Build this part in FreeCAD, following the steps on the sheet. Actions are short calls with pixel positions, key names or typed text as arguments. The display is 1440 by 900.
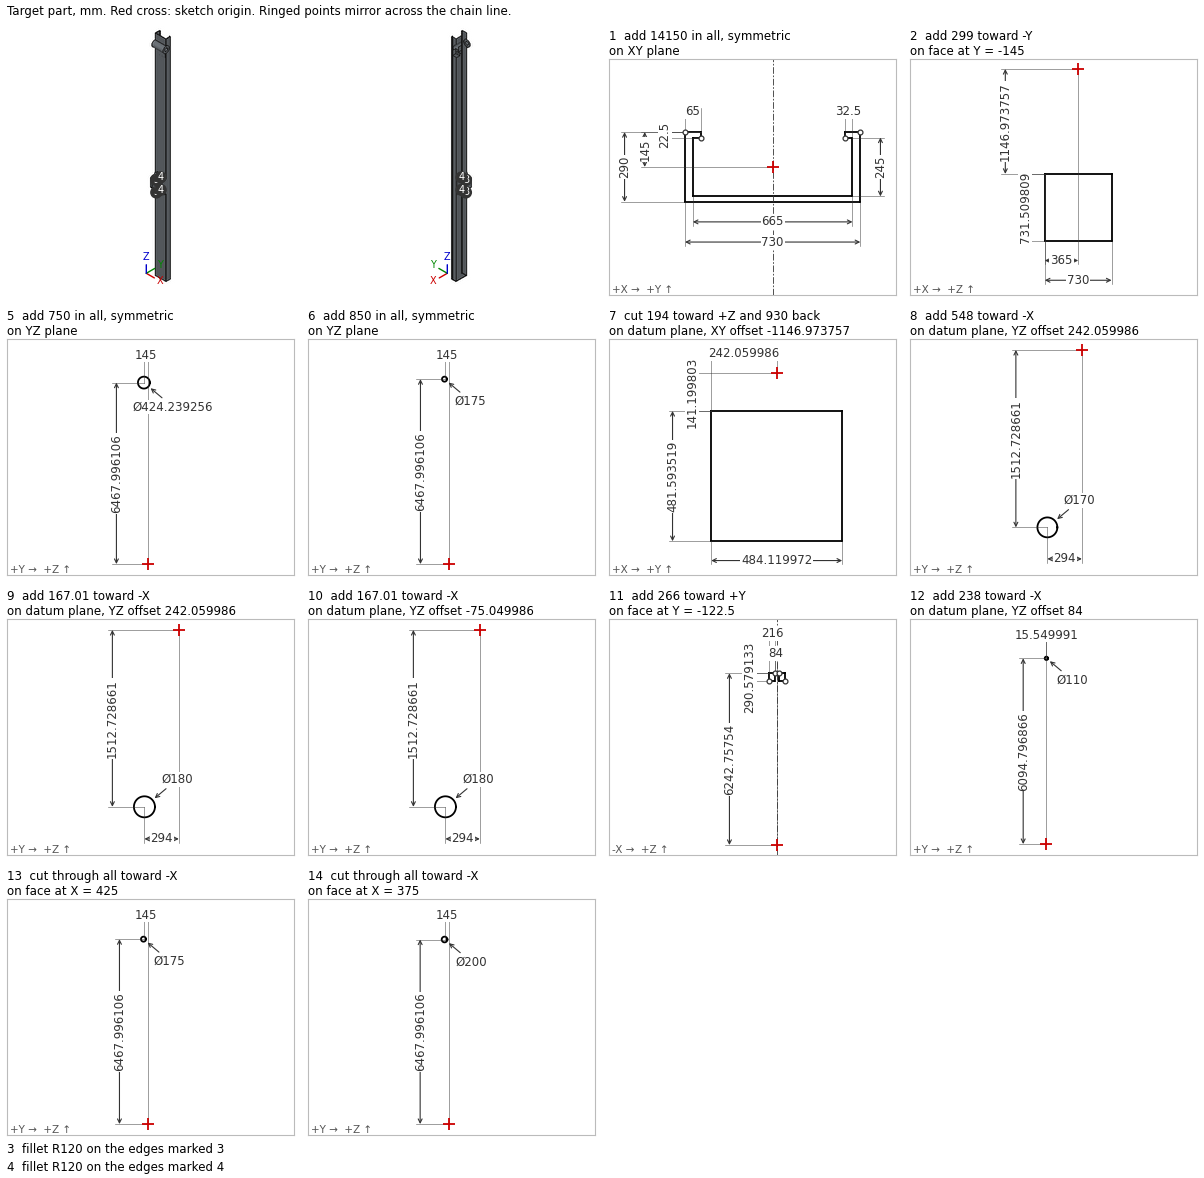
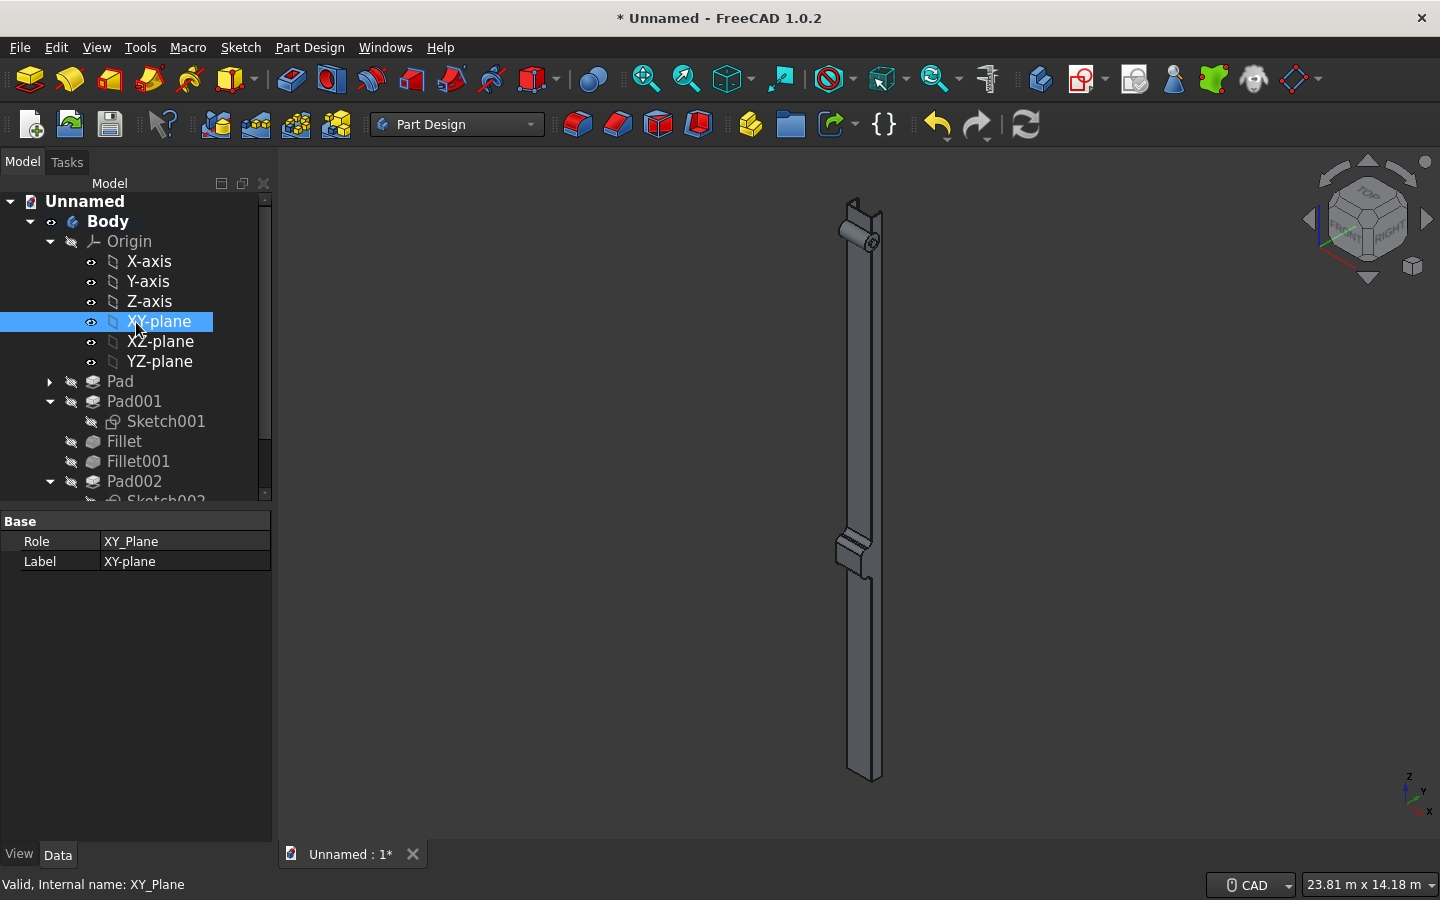
click(1294, 80)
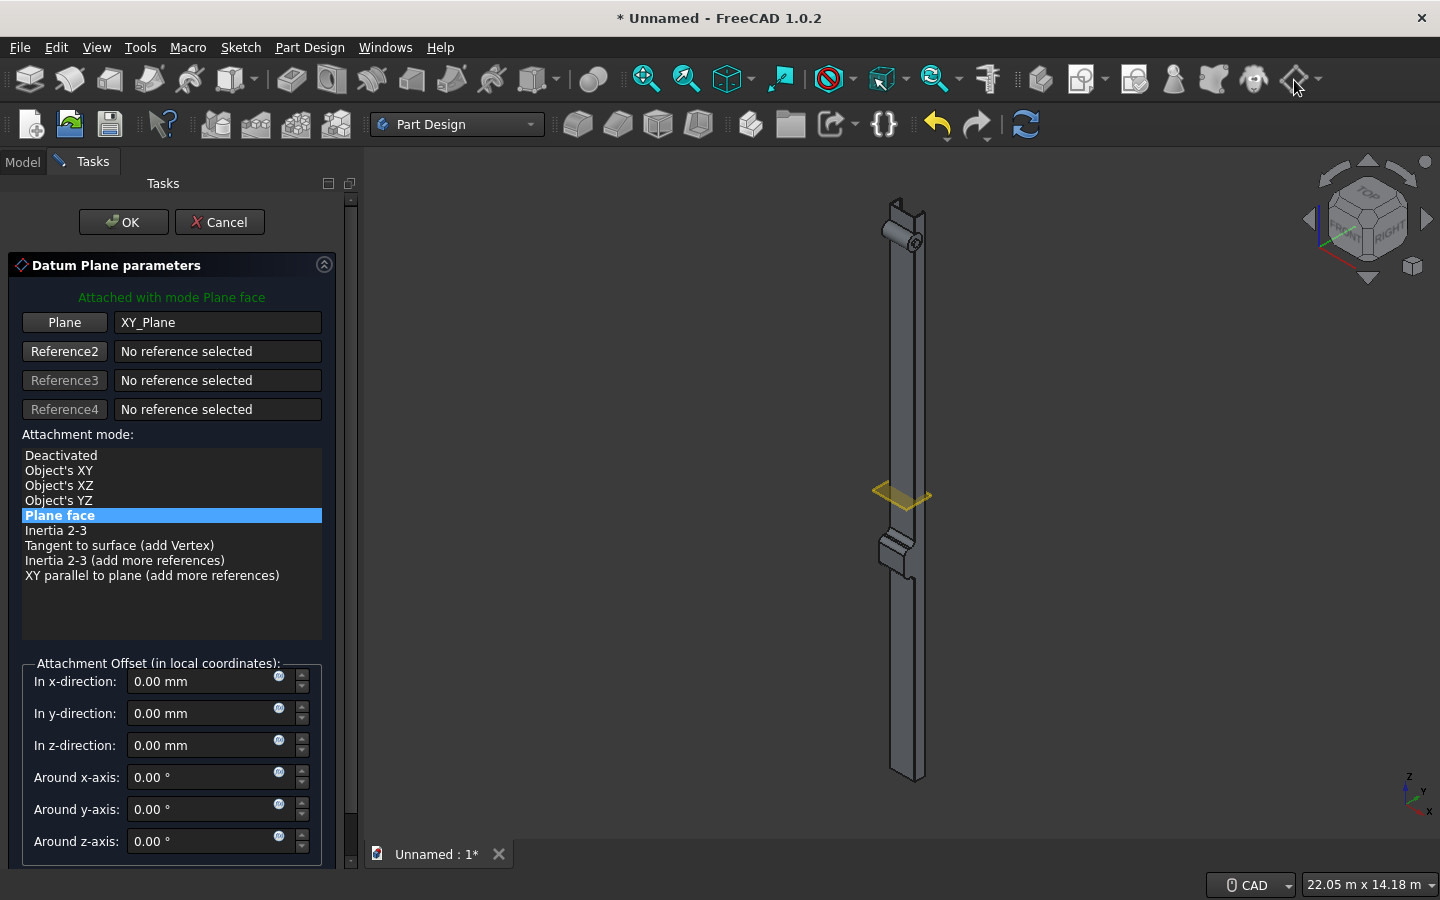
triple_click(210, 745)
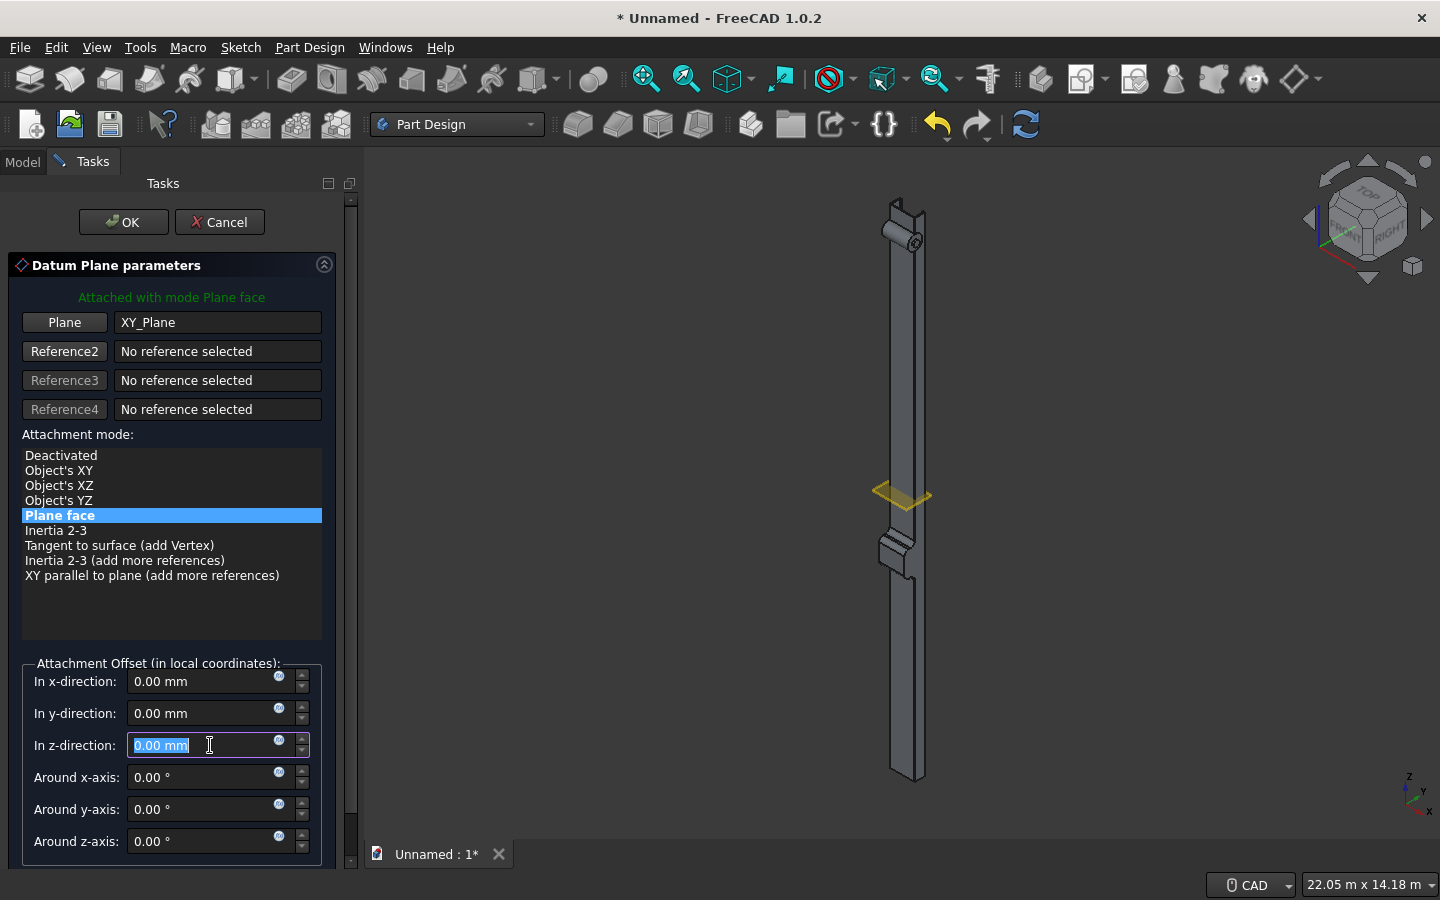
text(-1146.973757)
key(Tab)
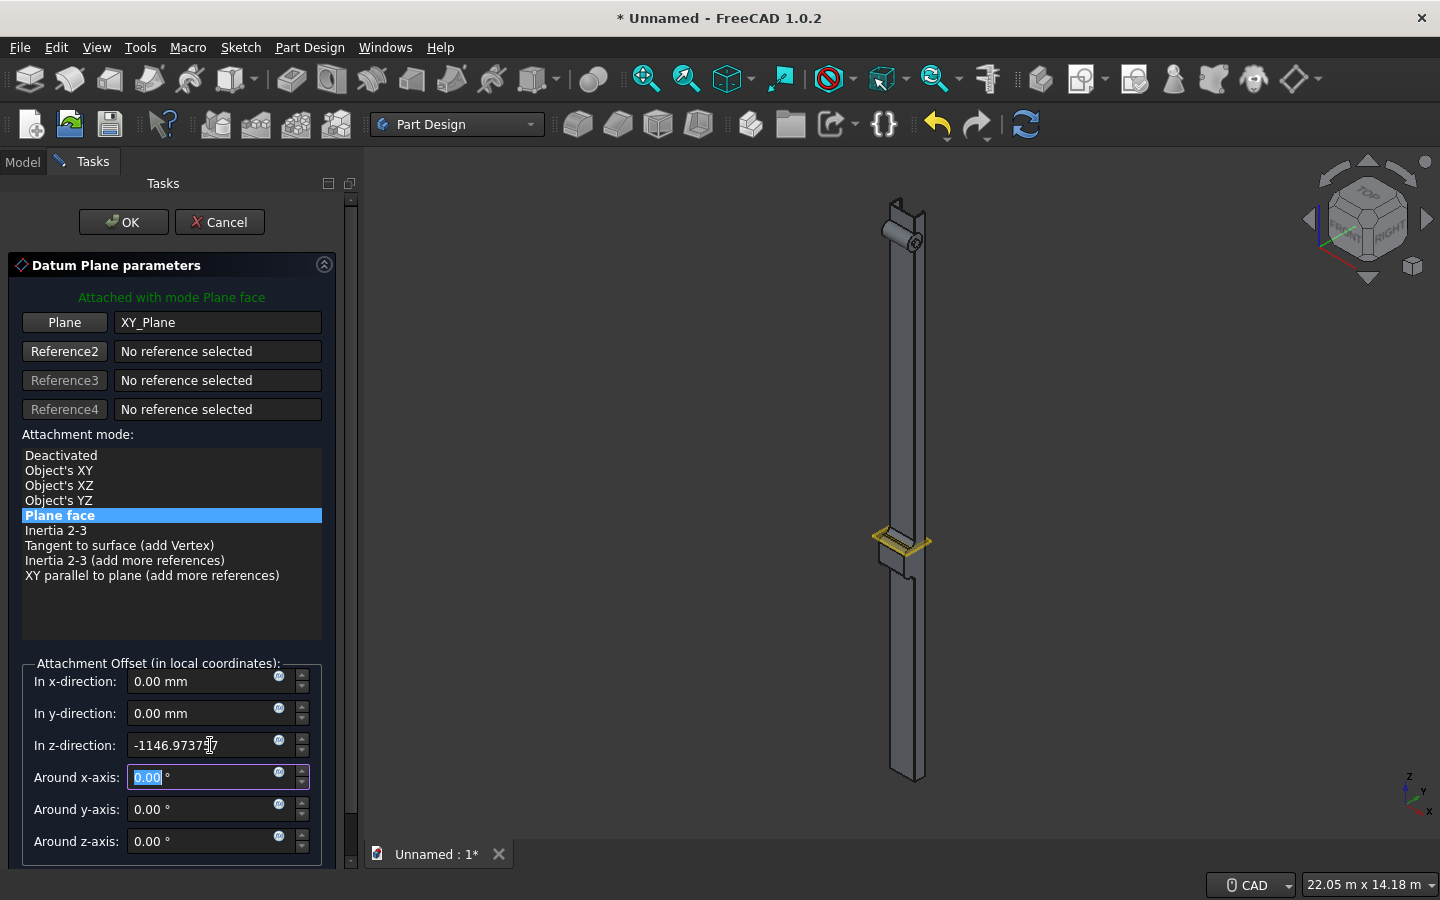
click(124, 222)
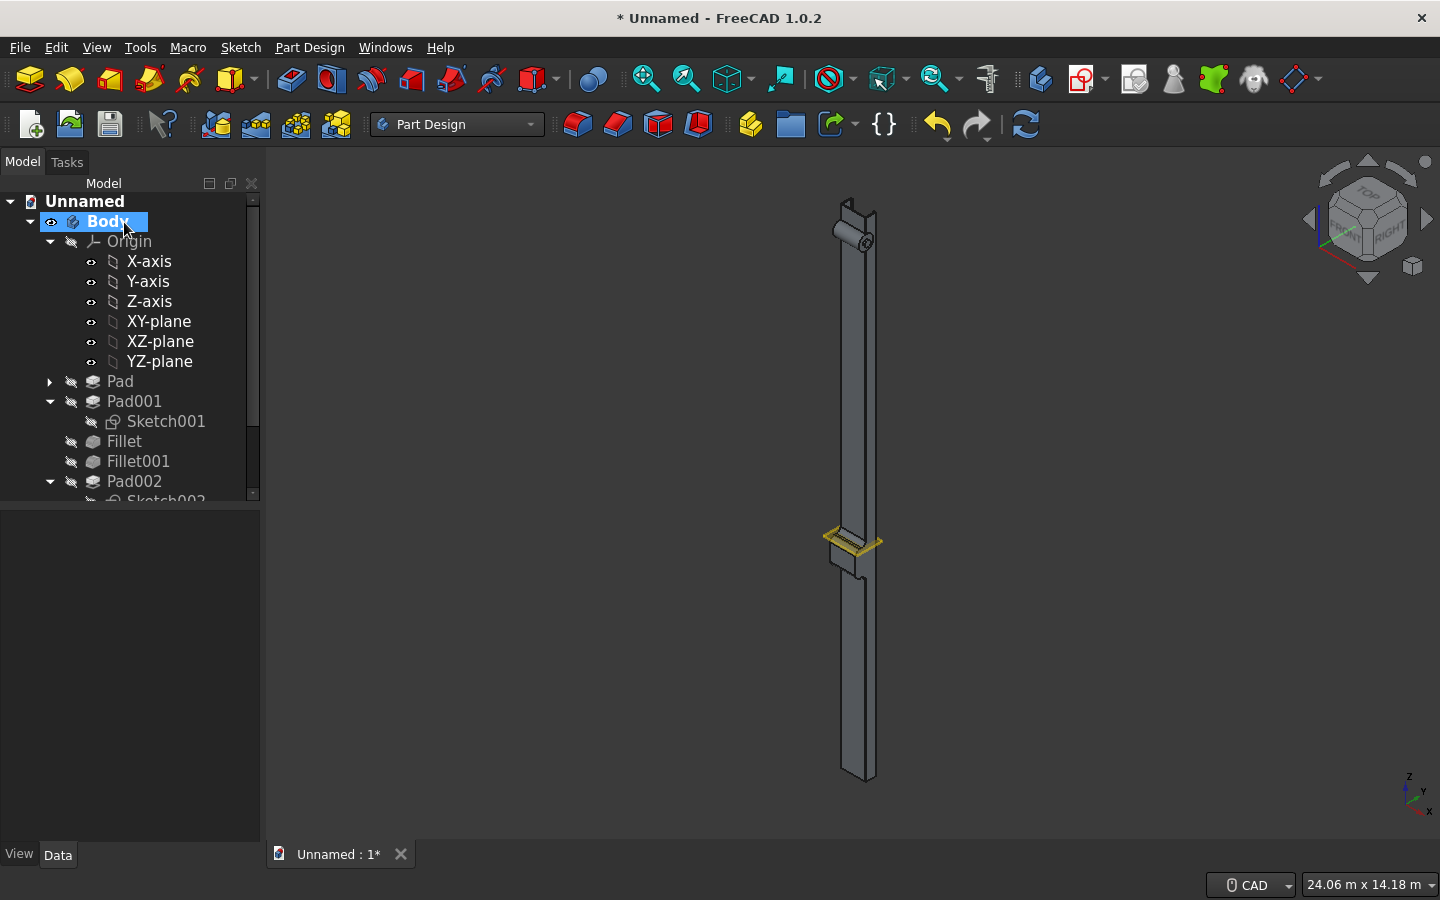
scroll(100, 337, down, 3)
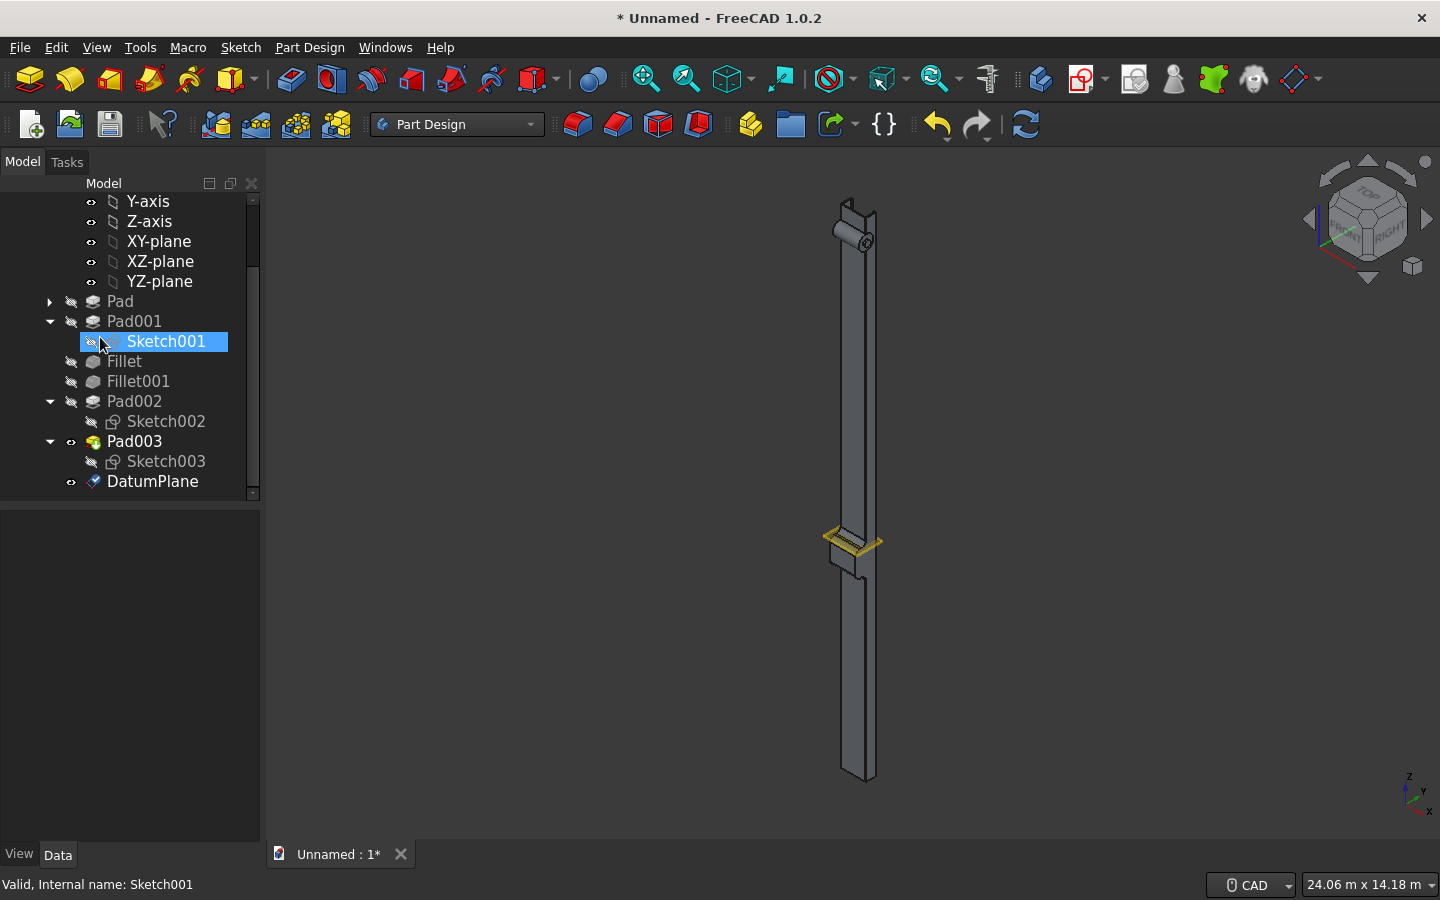
click(116, 482)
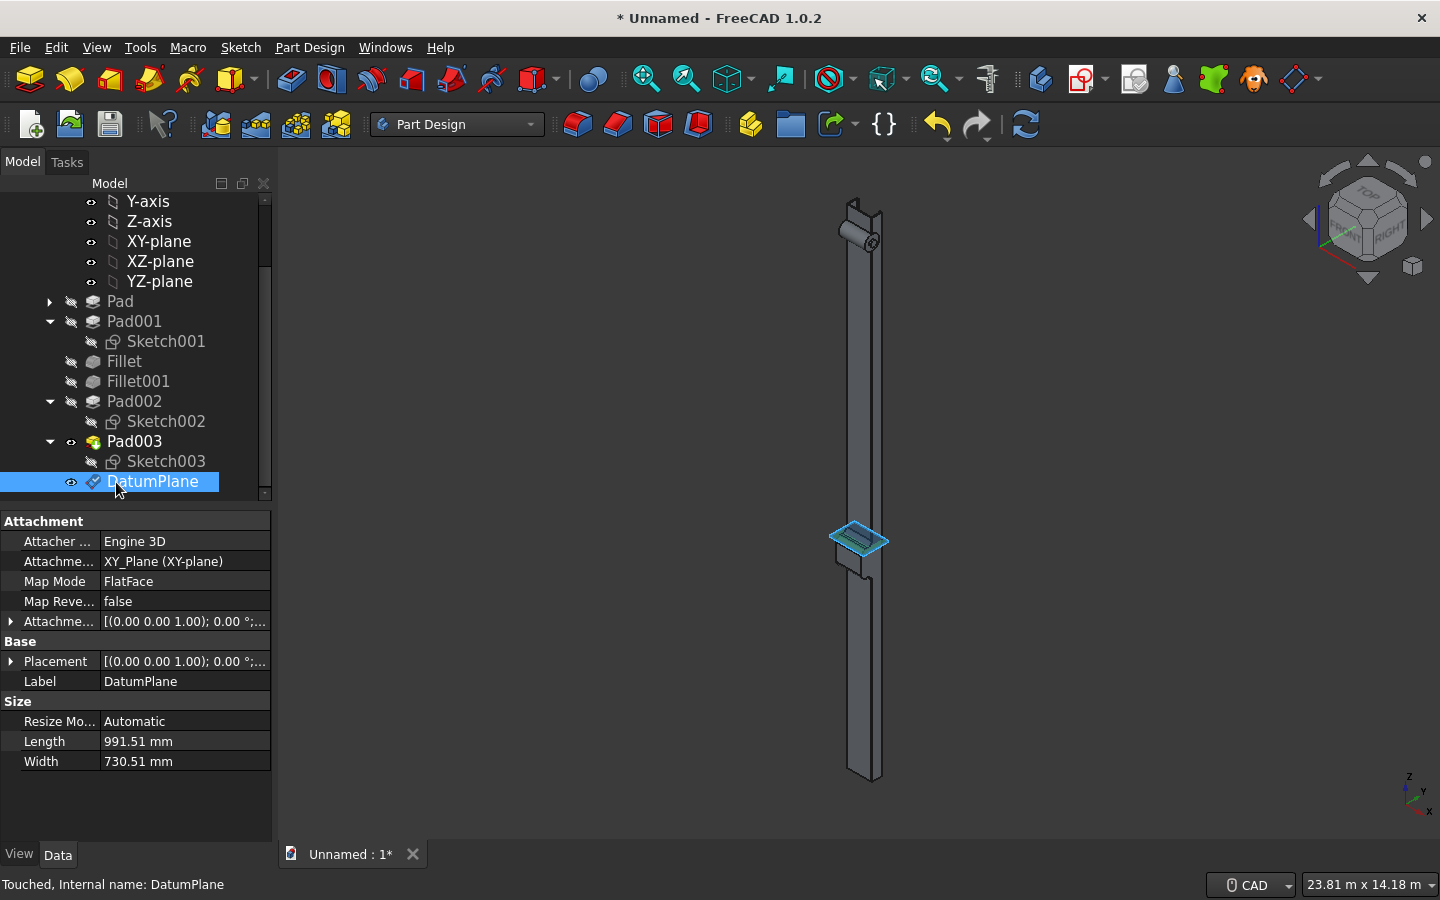
click(1082, 80)